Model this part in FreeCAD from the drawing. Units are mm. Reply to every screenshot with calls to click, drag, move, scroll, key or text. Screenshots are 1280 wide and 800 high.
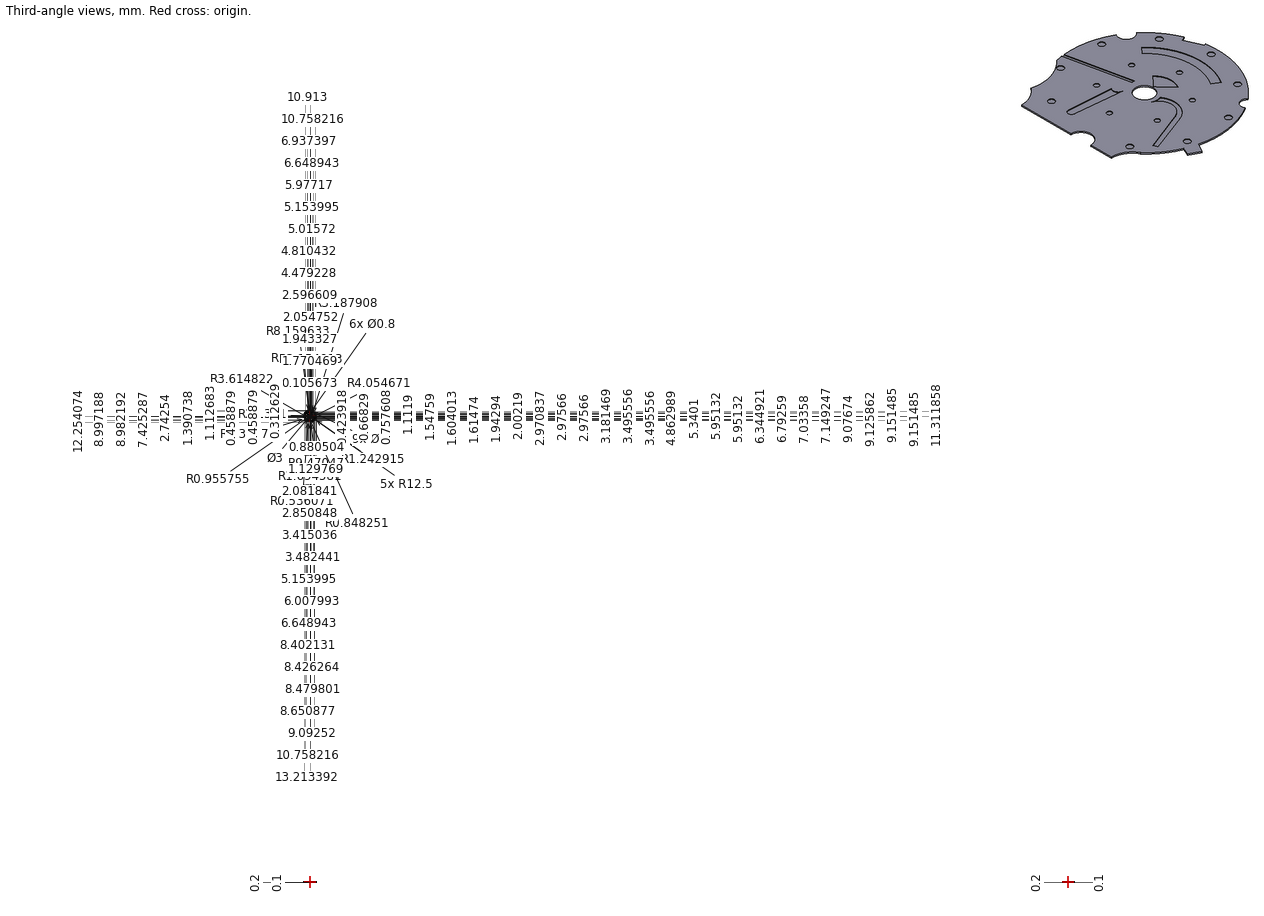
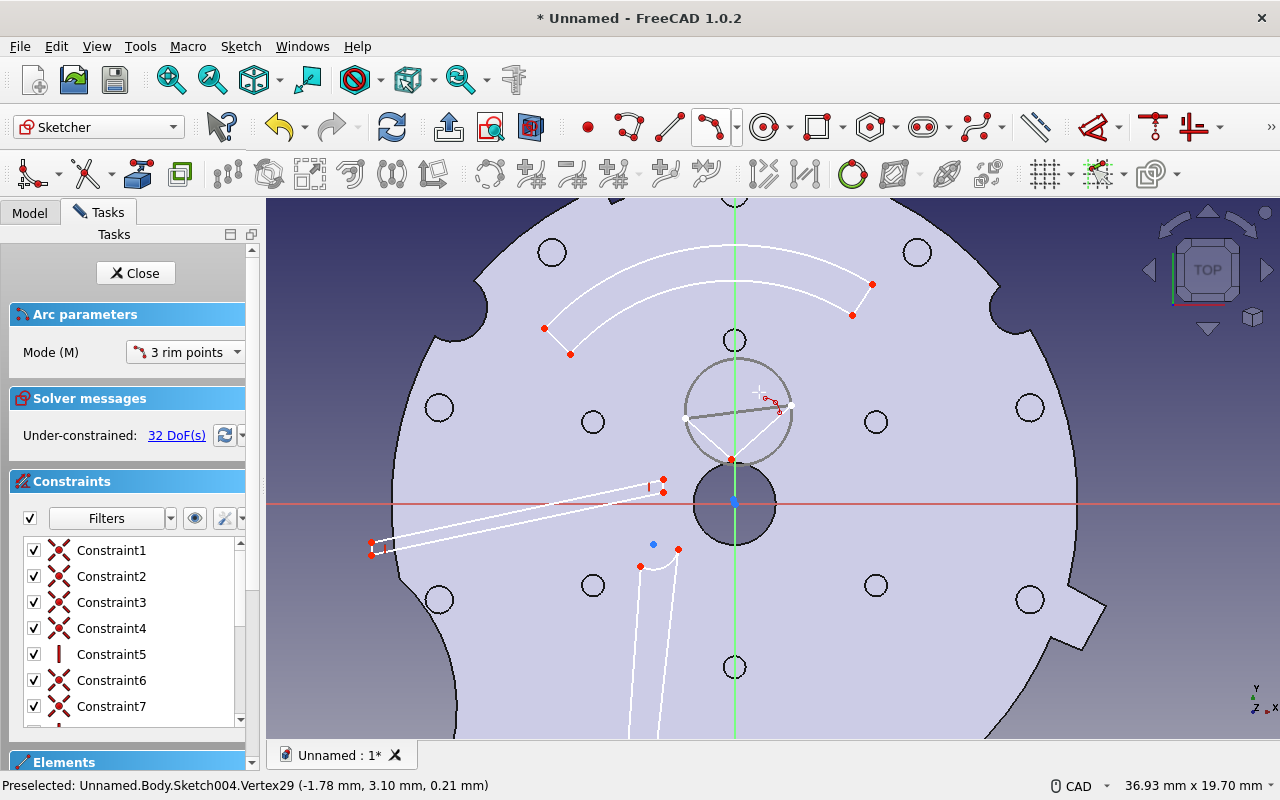
click(759, 391)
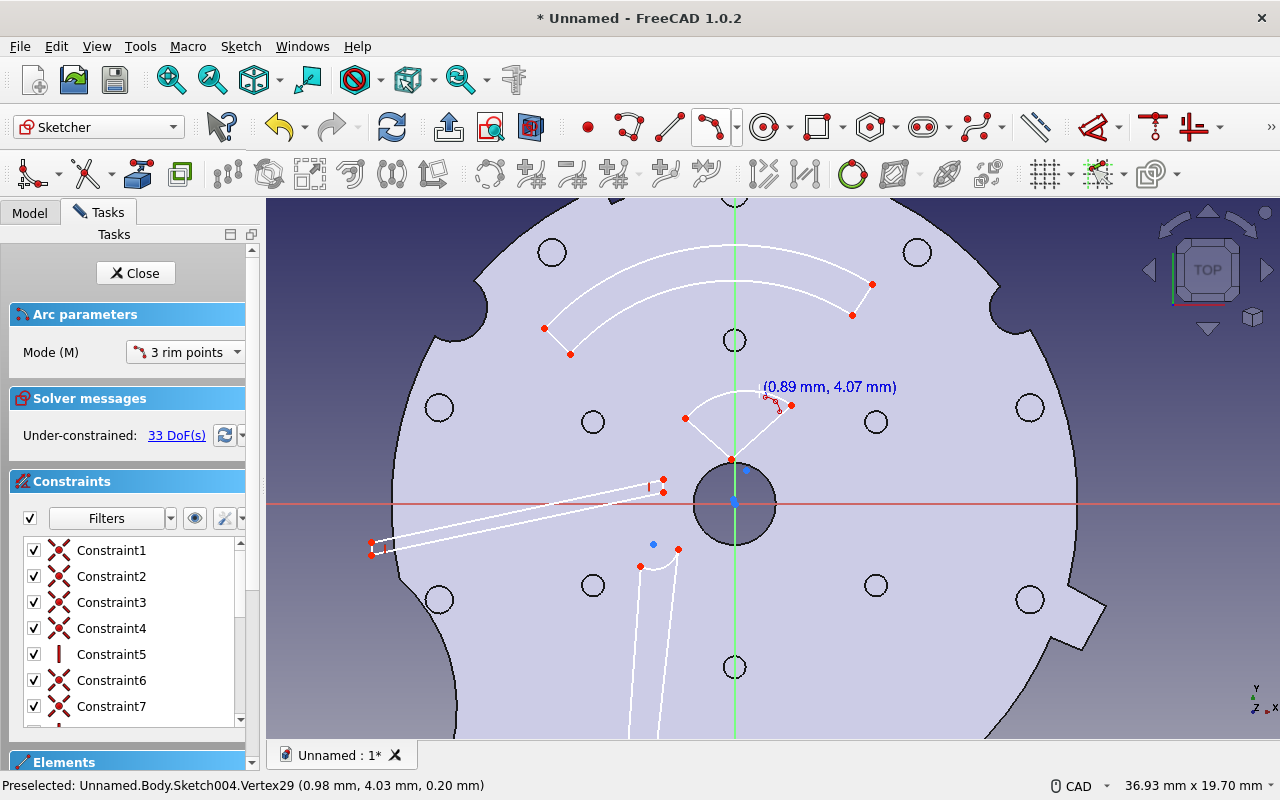
key(g)
key(m)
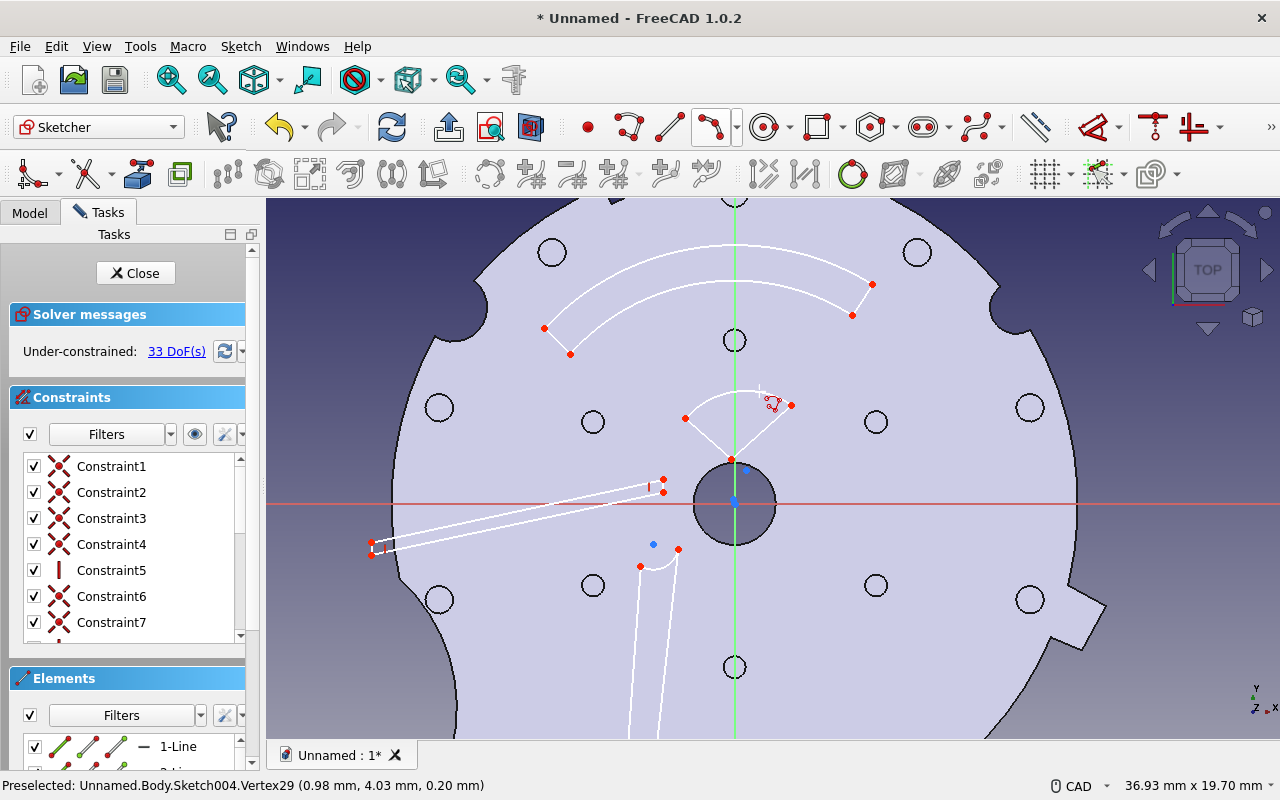
click(900, 525)
click(967, 697)
click(984, 690)
click(922, 526)
right_click(922, 526)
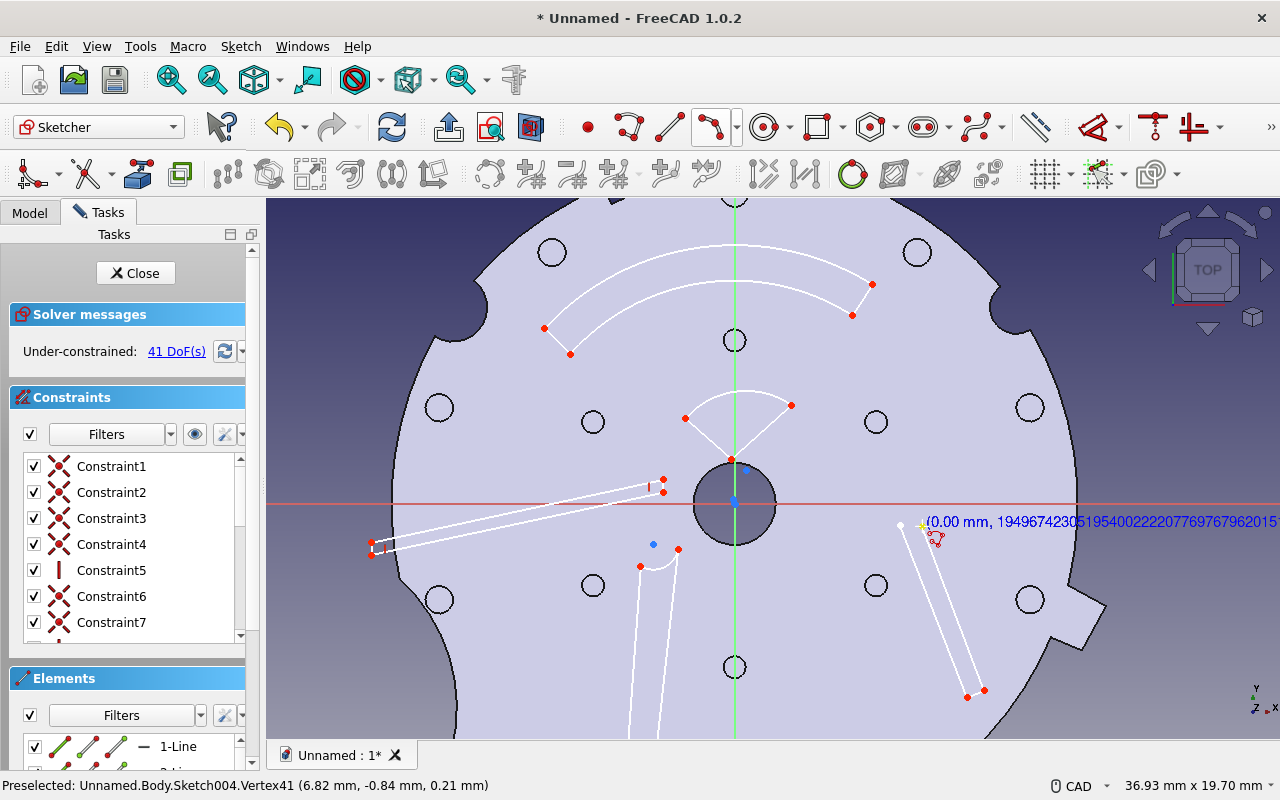
click(710, 128)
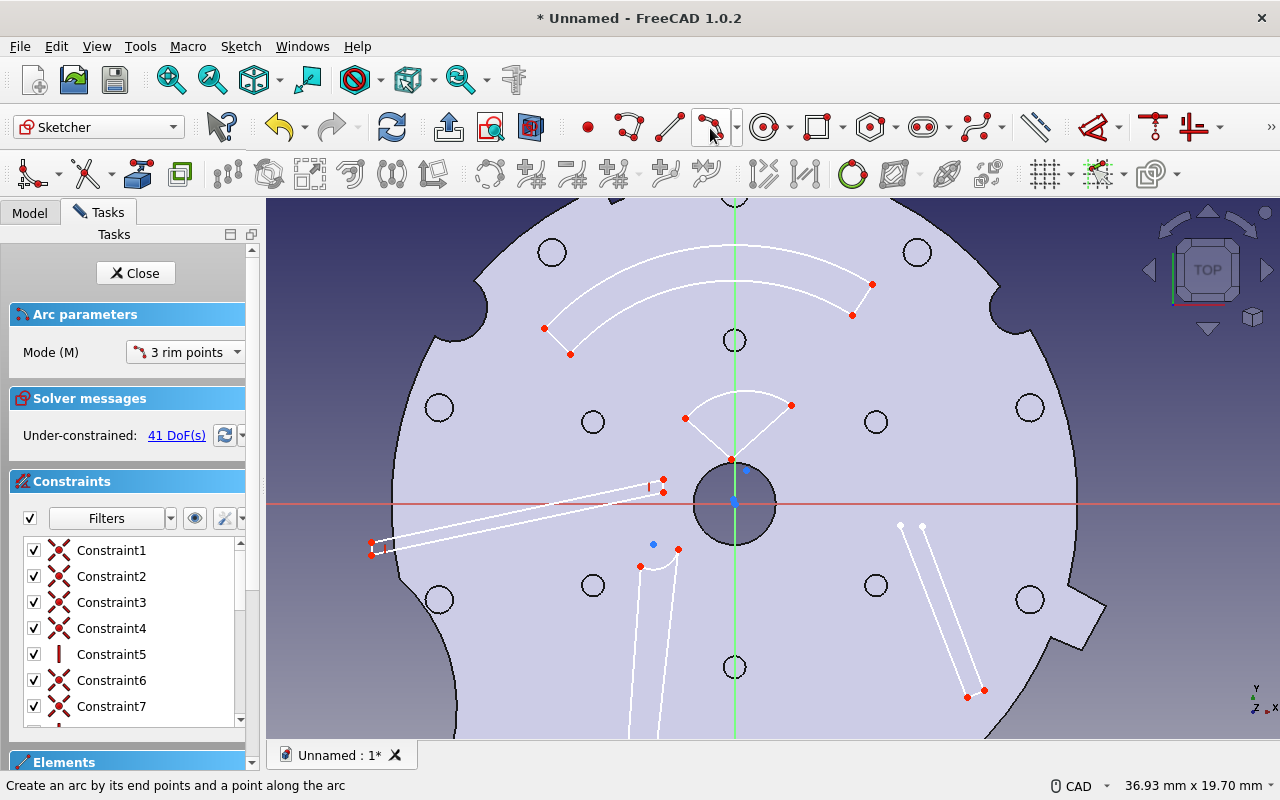
click(922, 527)
click(790, 485)
click(866, 474)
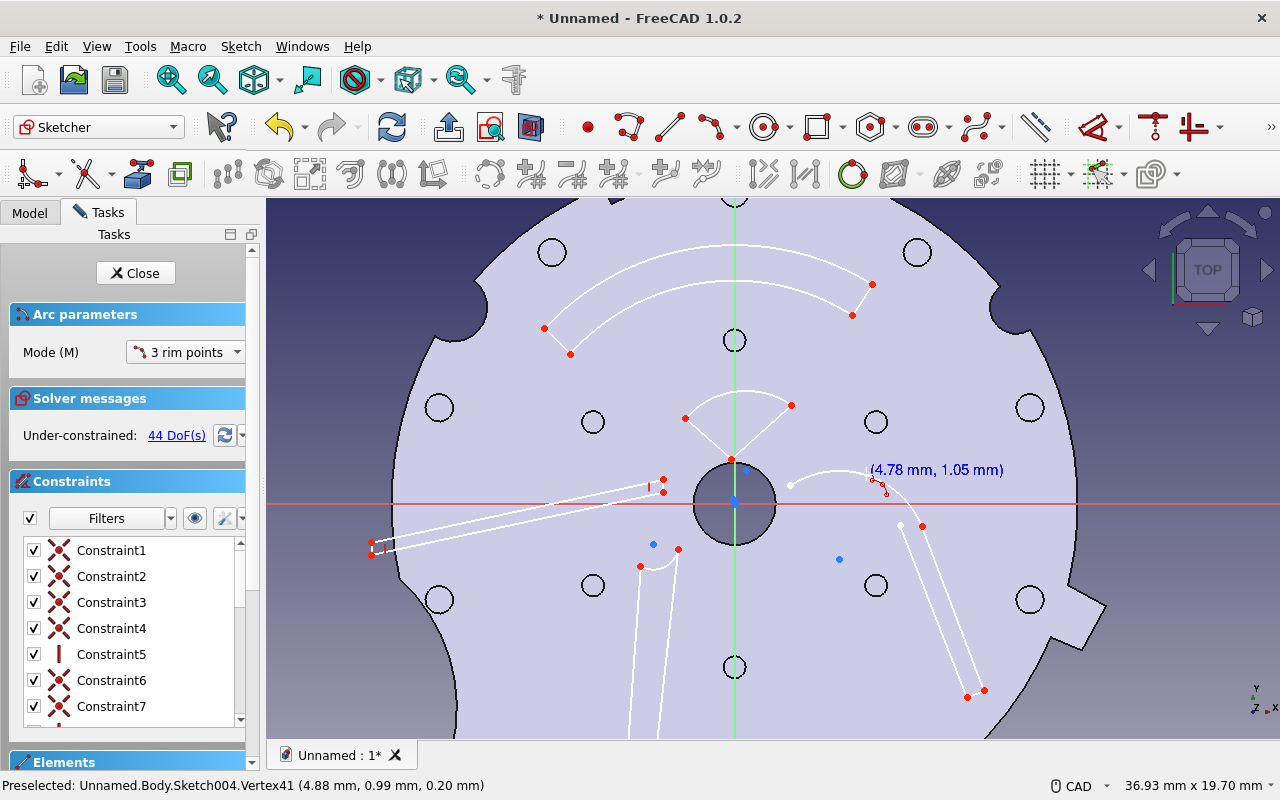
click(790, 486)
click(789, 525)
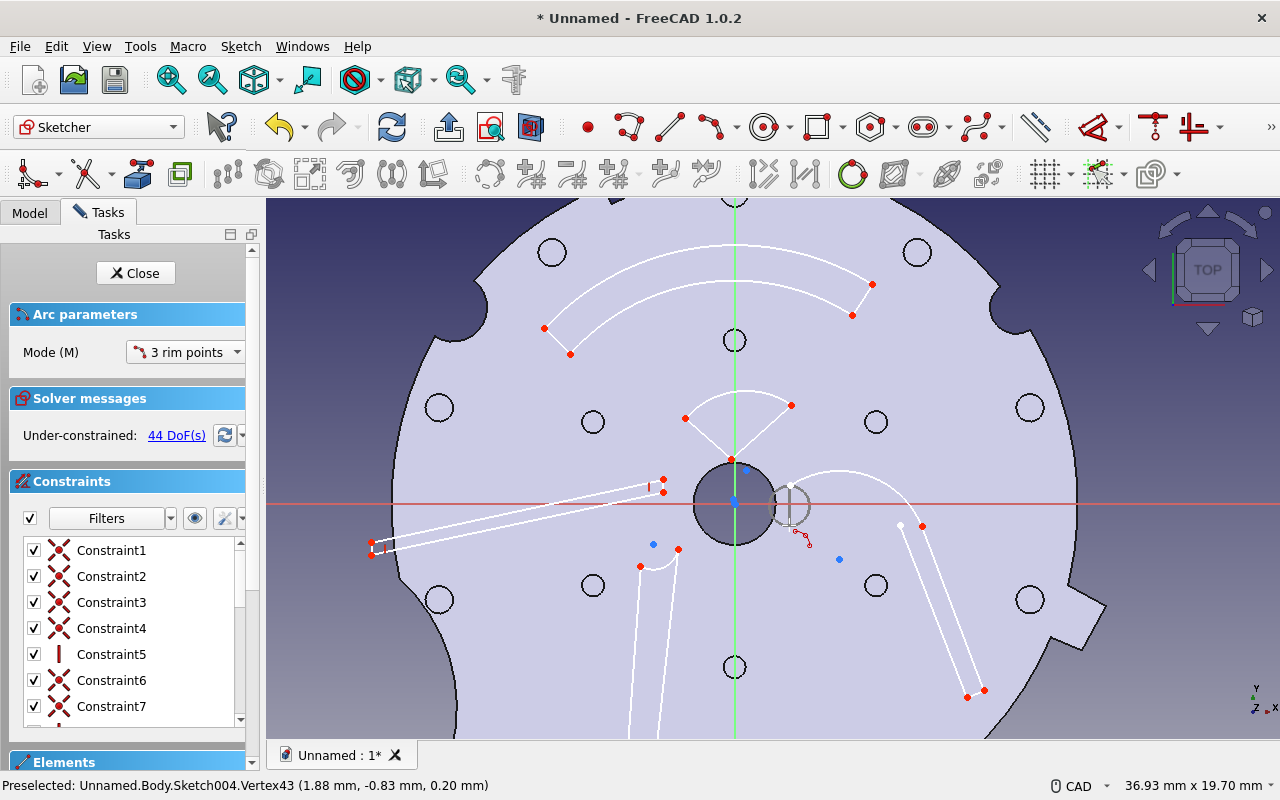
scroll(793, 509, up, 8)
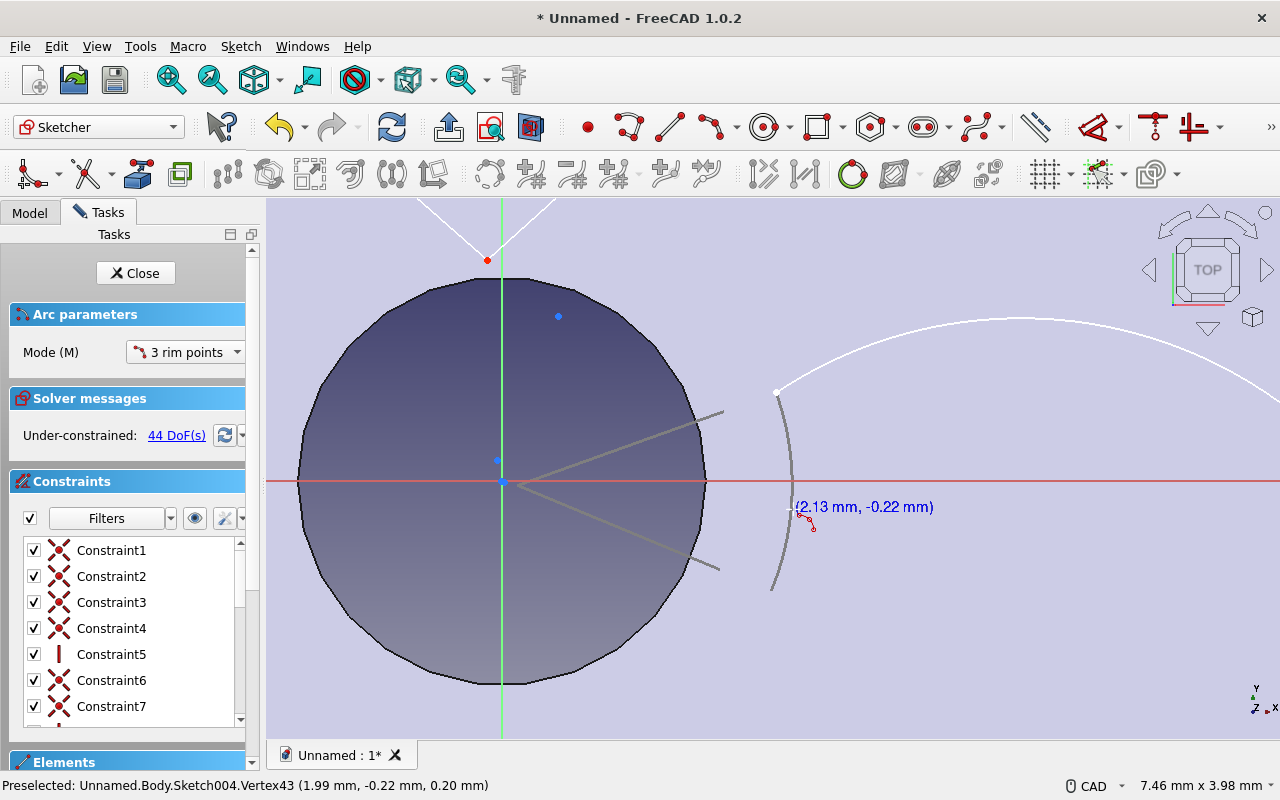
click(791, 508)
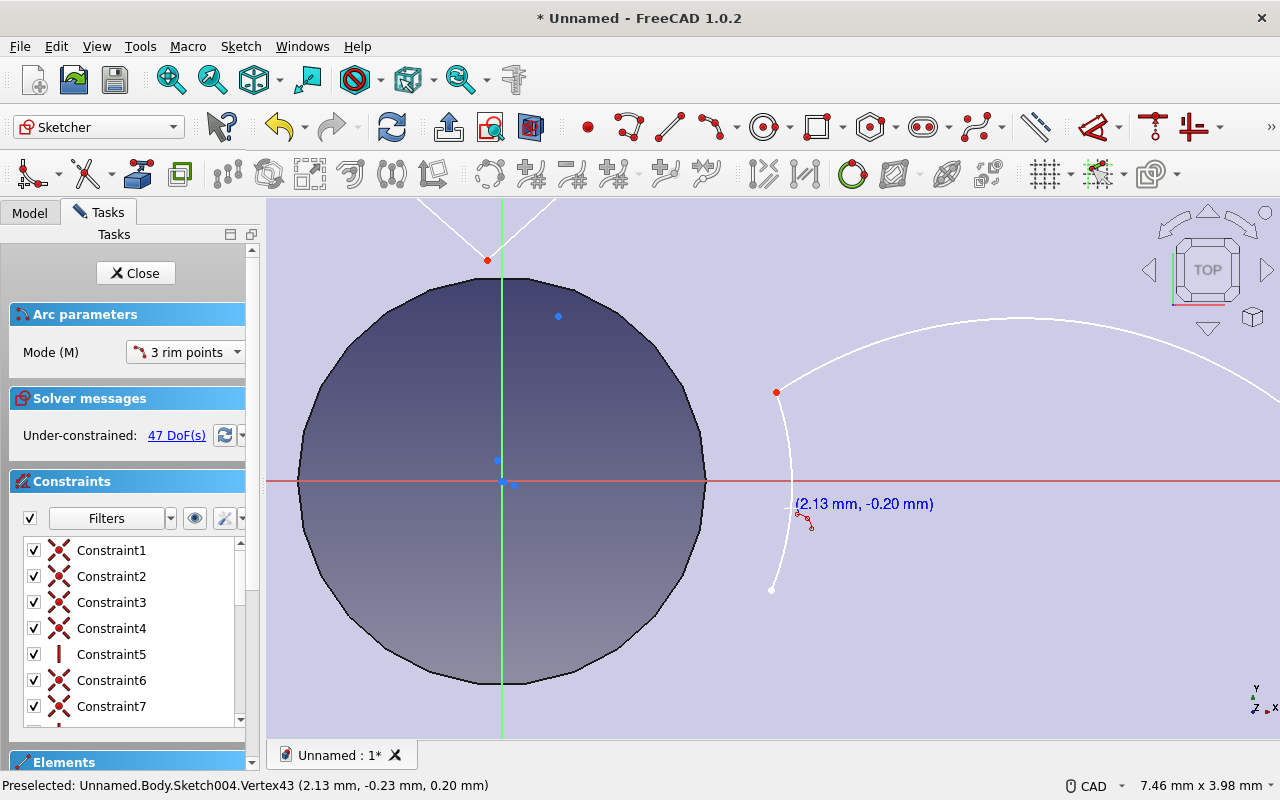
scroll(780, 465, down, 10)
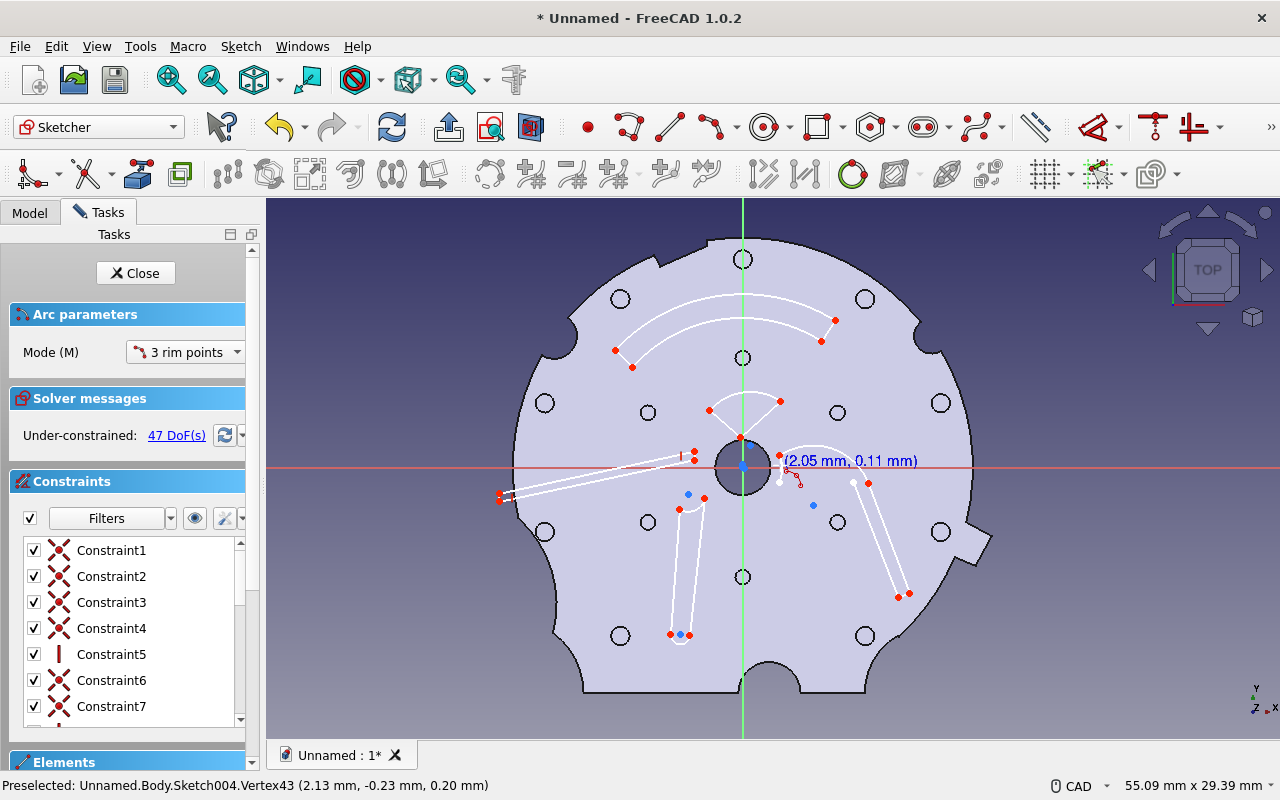
click(779, 482)
click(854, 482)